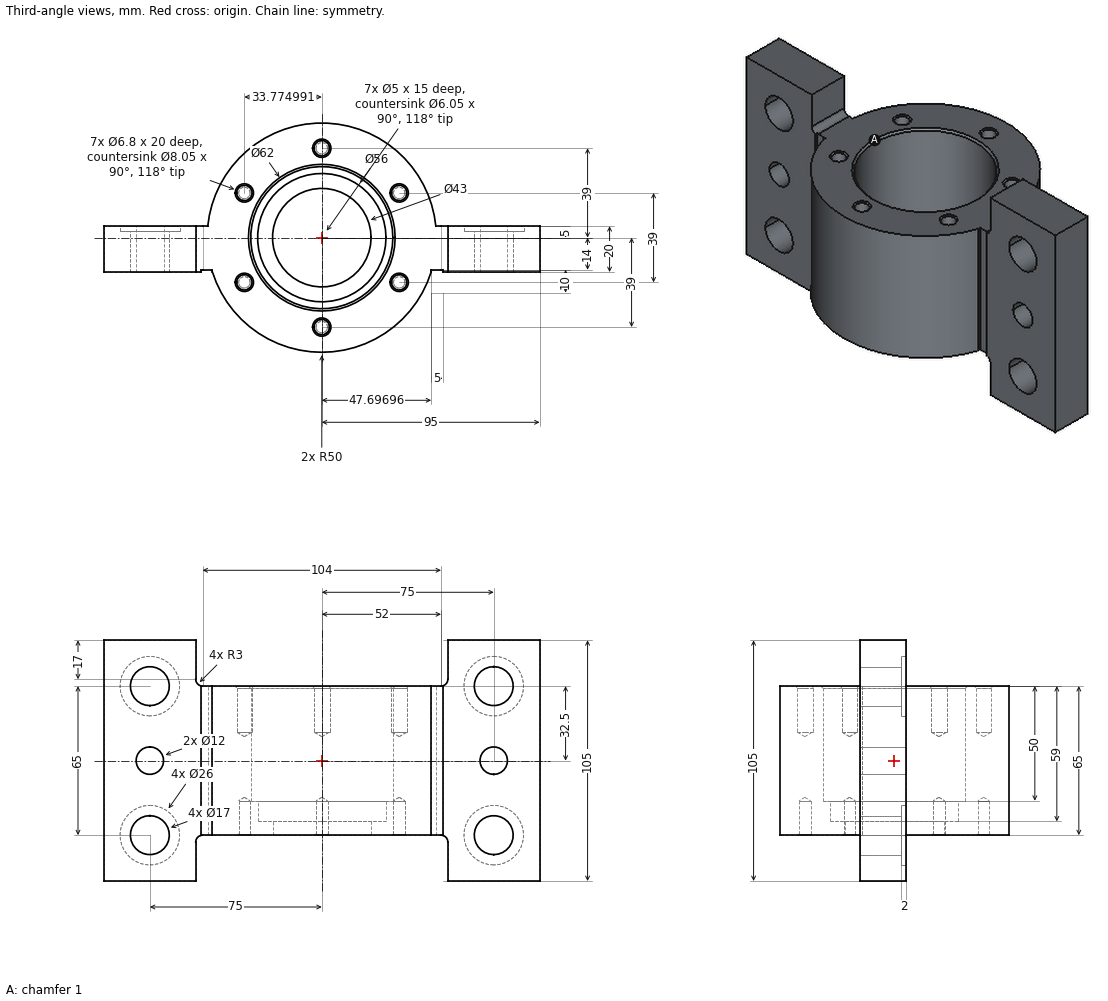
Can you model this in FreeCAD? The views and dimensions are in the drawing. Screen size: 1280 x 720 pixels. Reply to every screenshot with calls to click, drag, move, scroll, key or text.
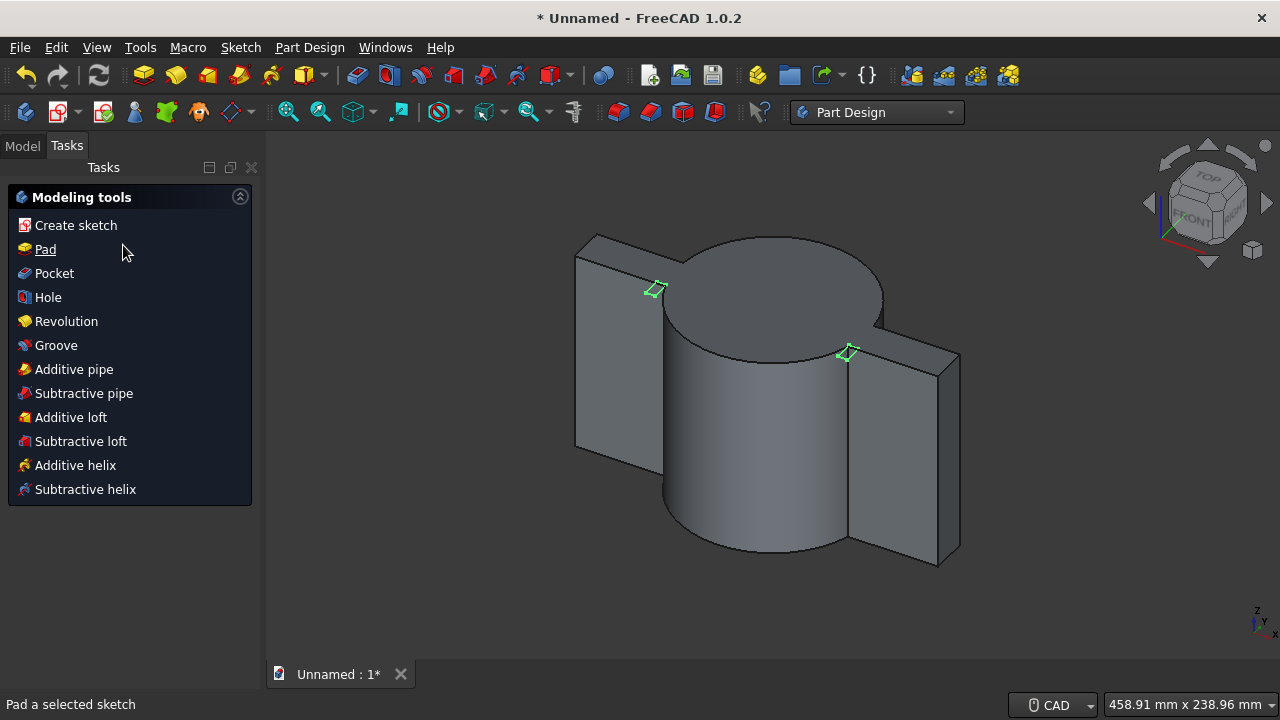
click(358, 76)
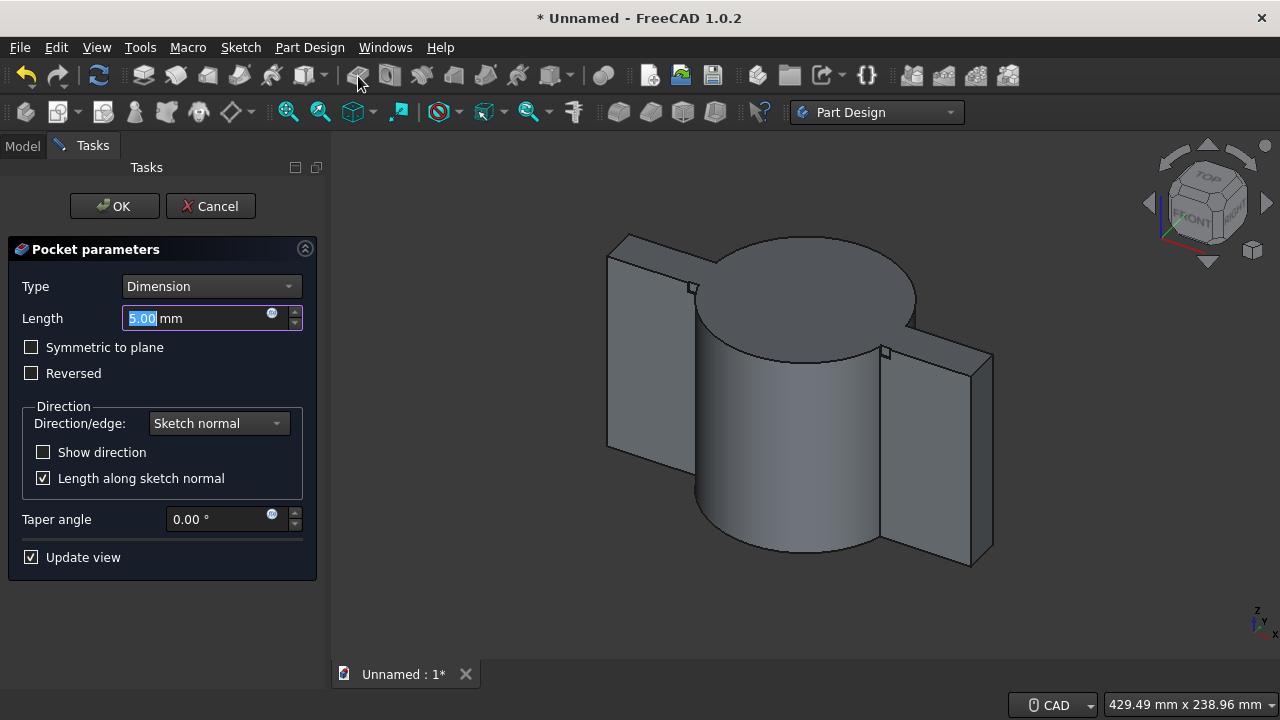
text(105)
key(Tab)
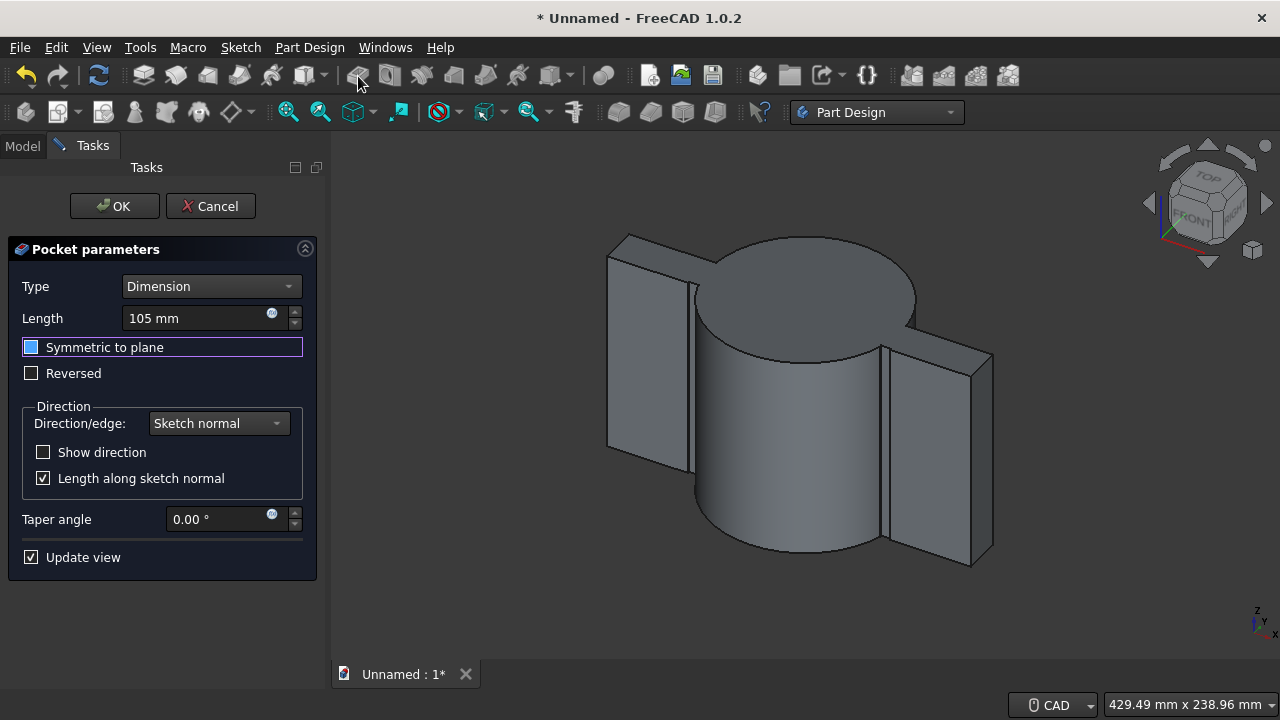
click(115, 206)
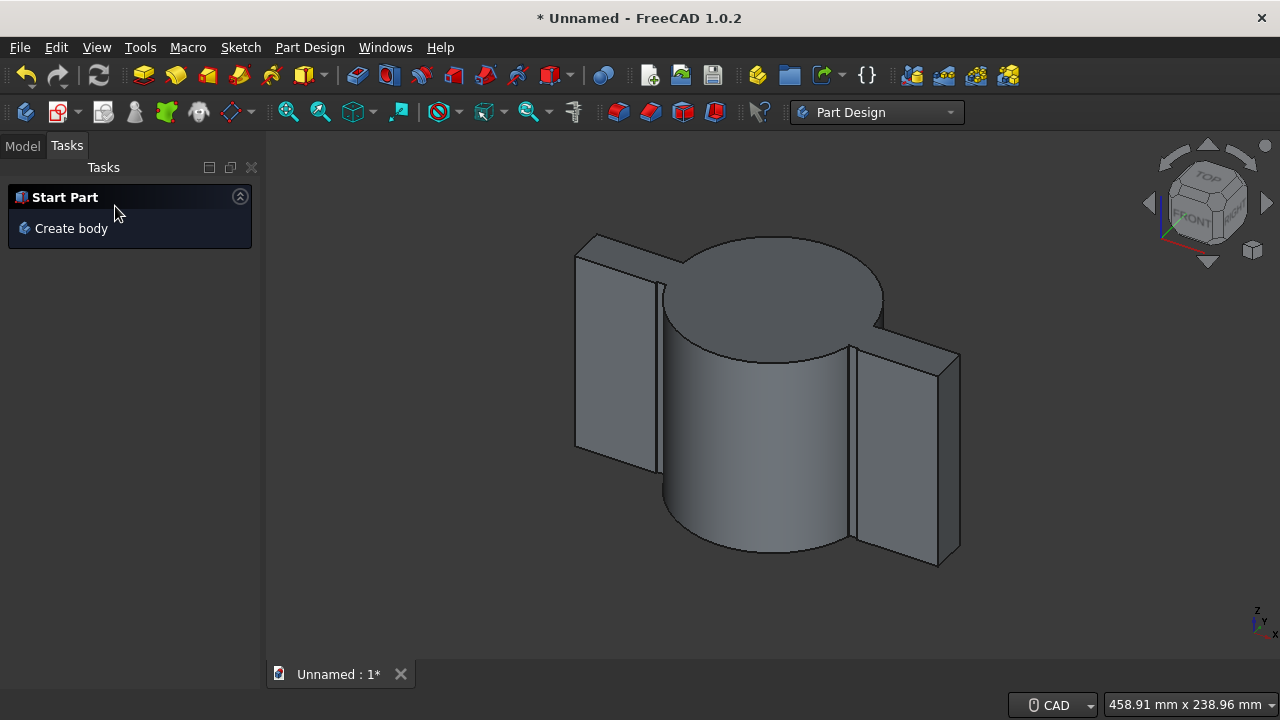
key(4)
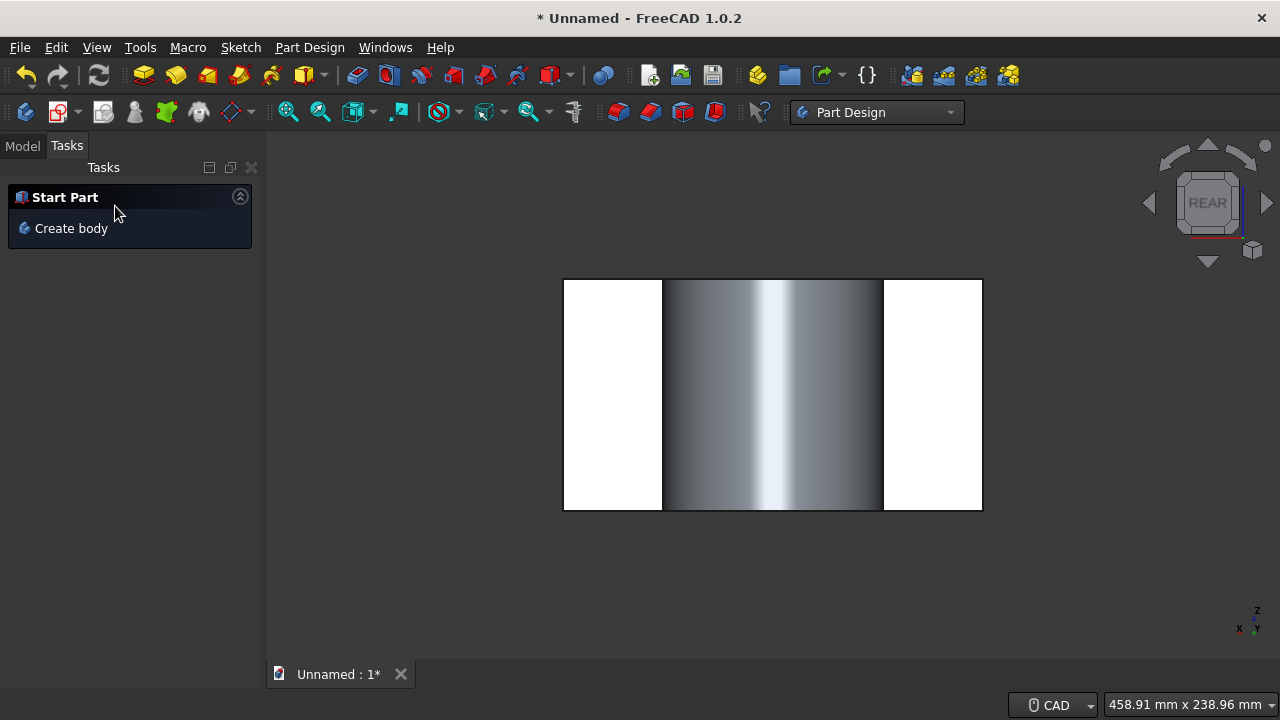
click(290, 112)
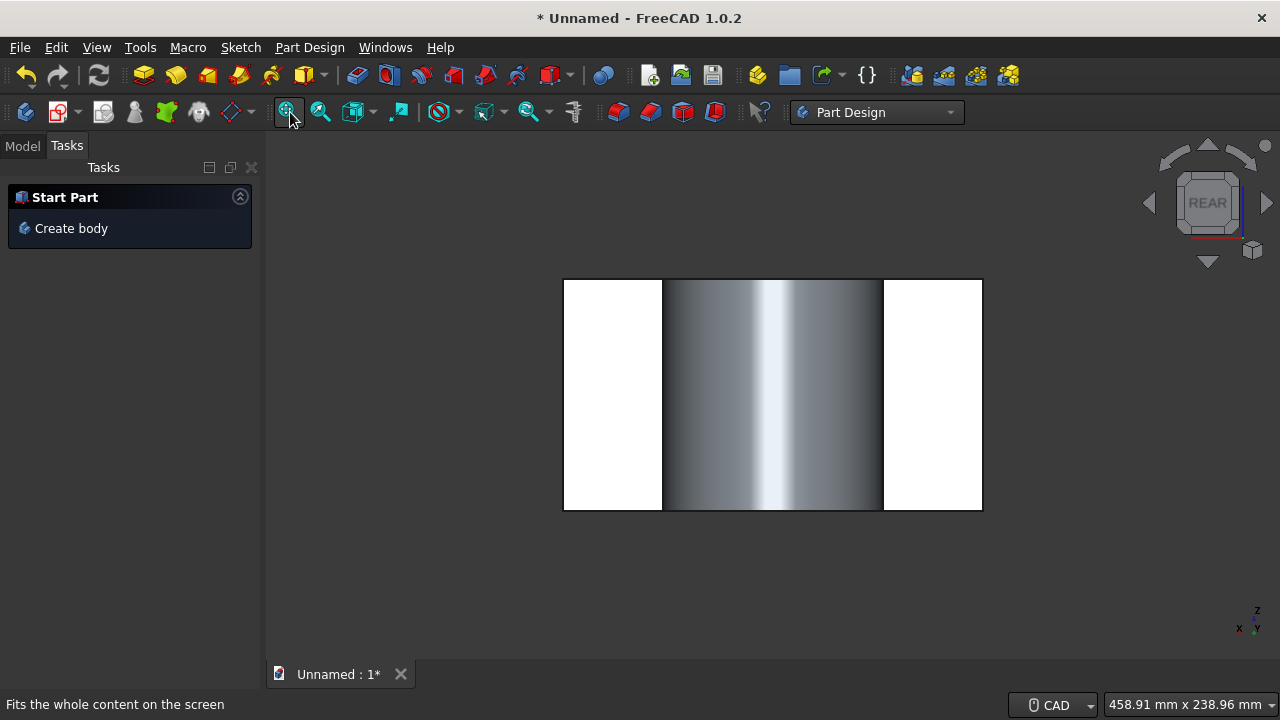
click(613, 361)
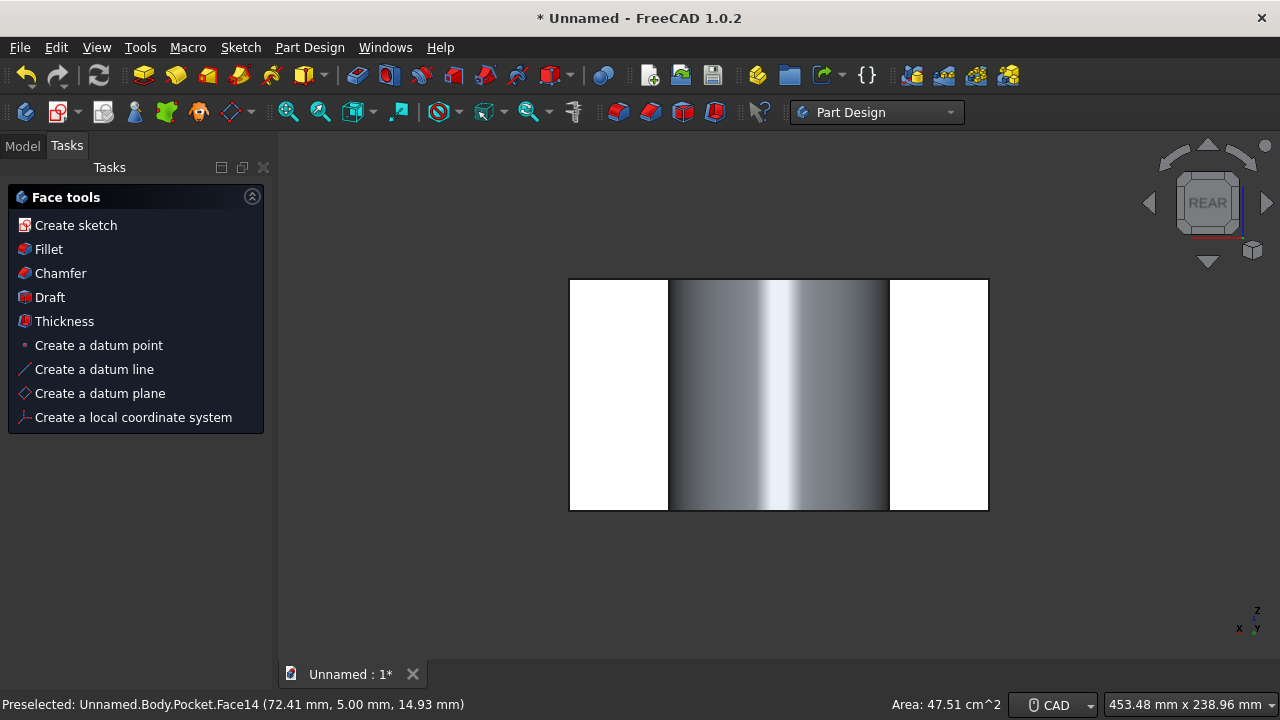
click(58, 112)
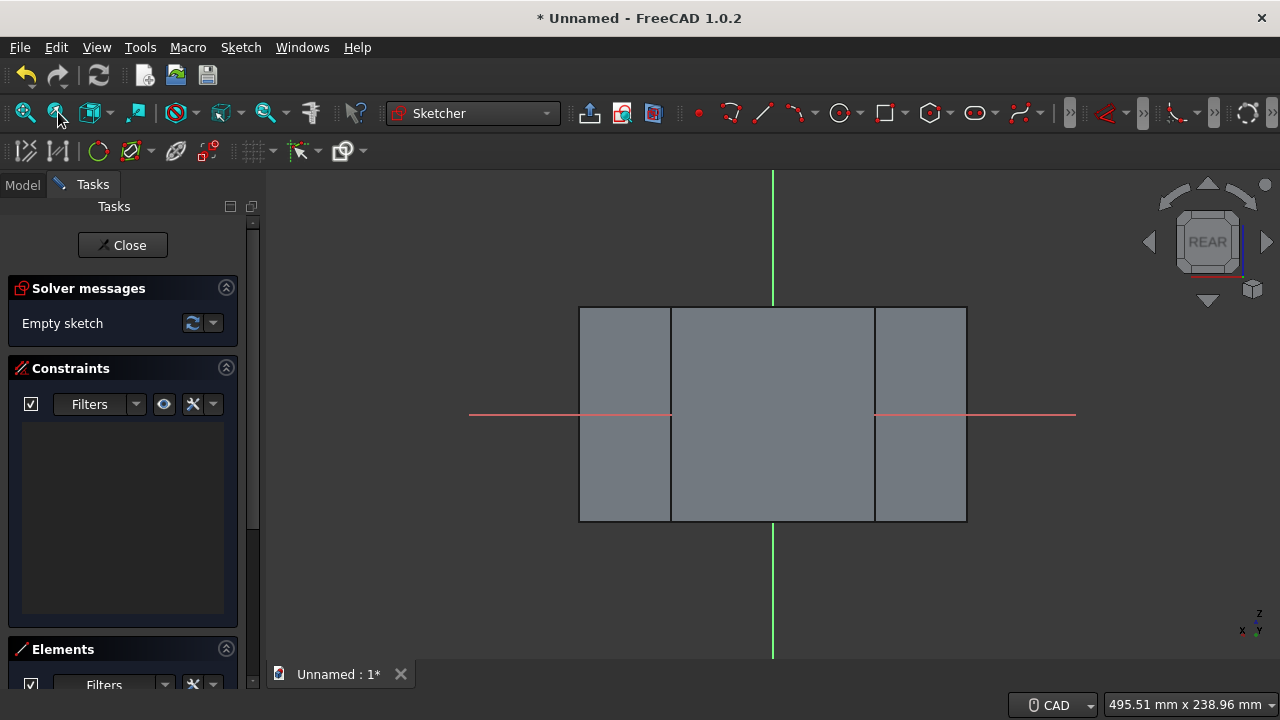
scroll(912, 414, up, 2)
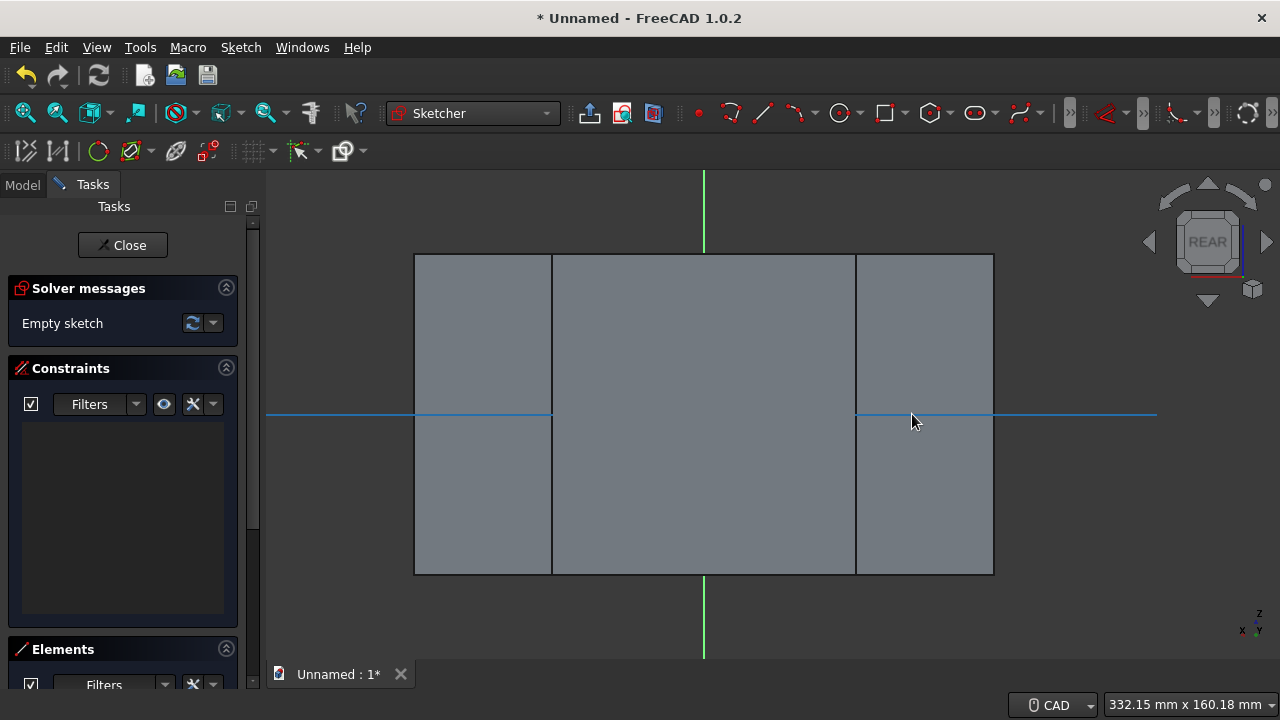
click(764, 114)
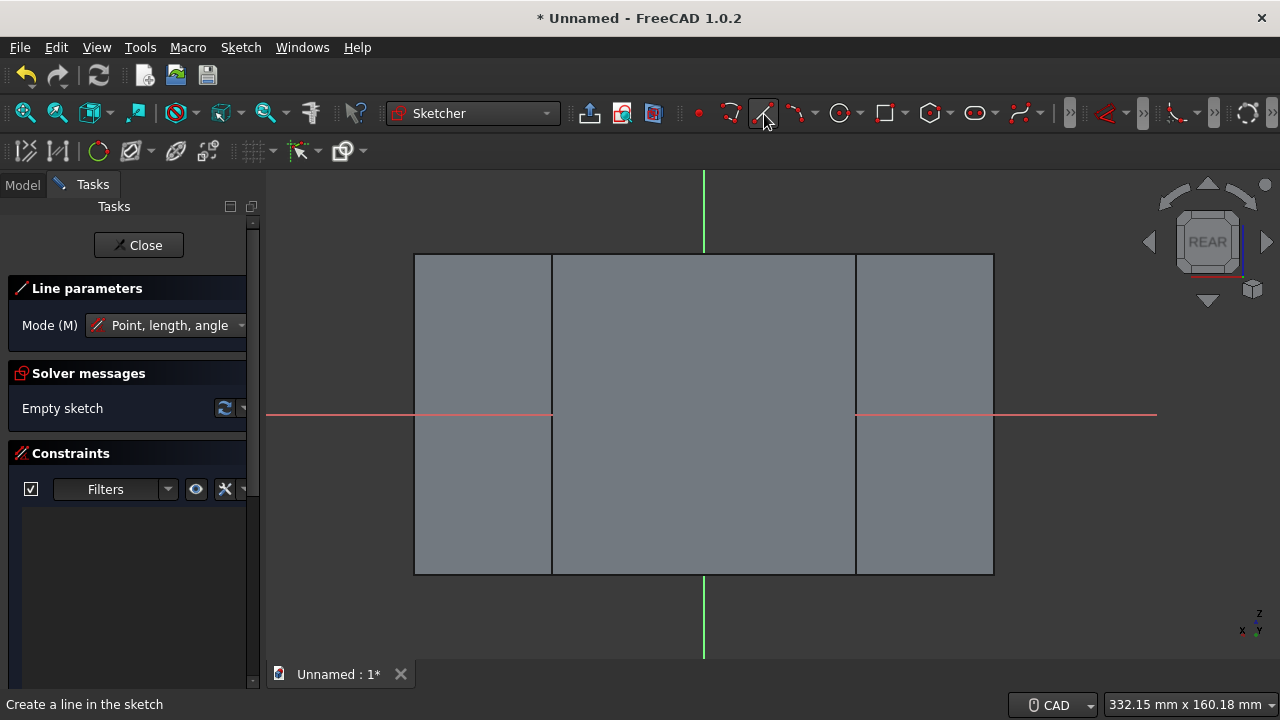
click(546, 315)
click(863, 315)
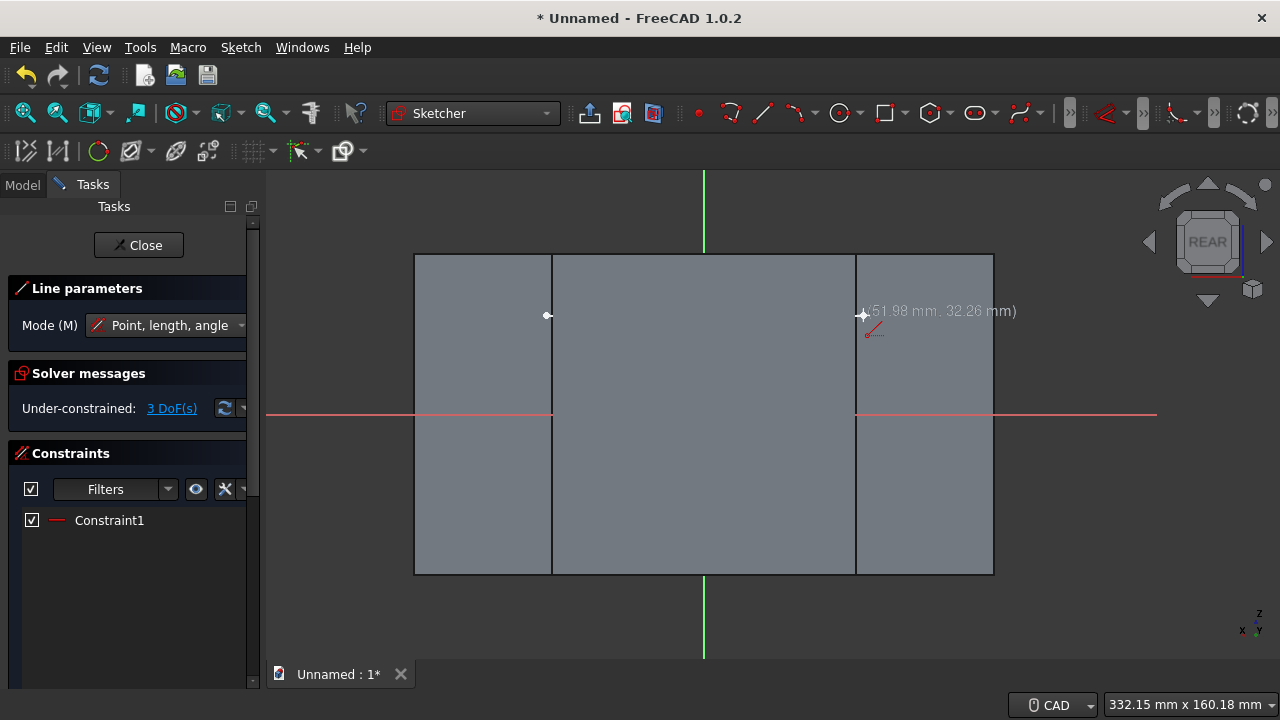
click(732, 114)